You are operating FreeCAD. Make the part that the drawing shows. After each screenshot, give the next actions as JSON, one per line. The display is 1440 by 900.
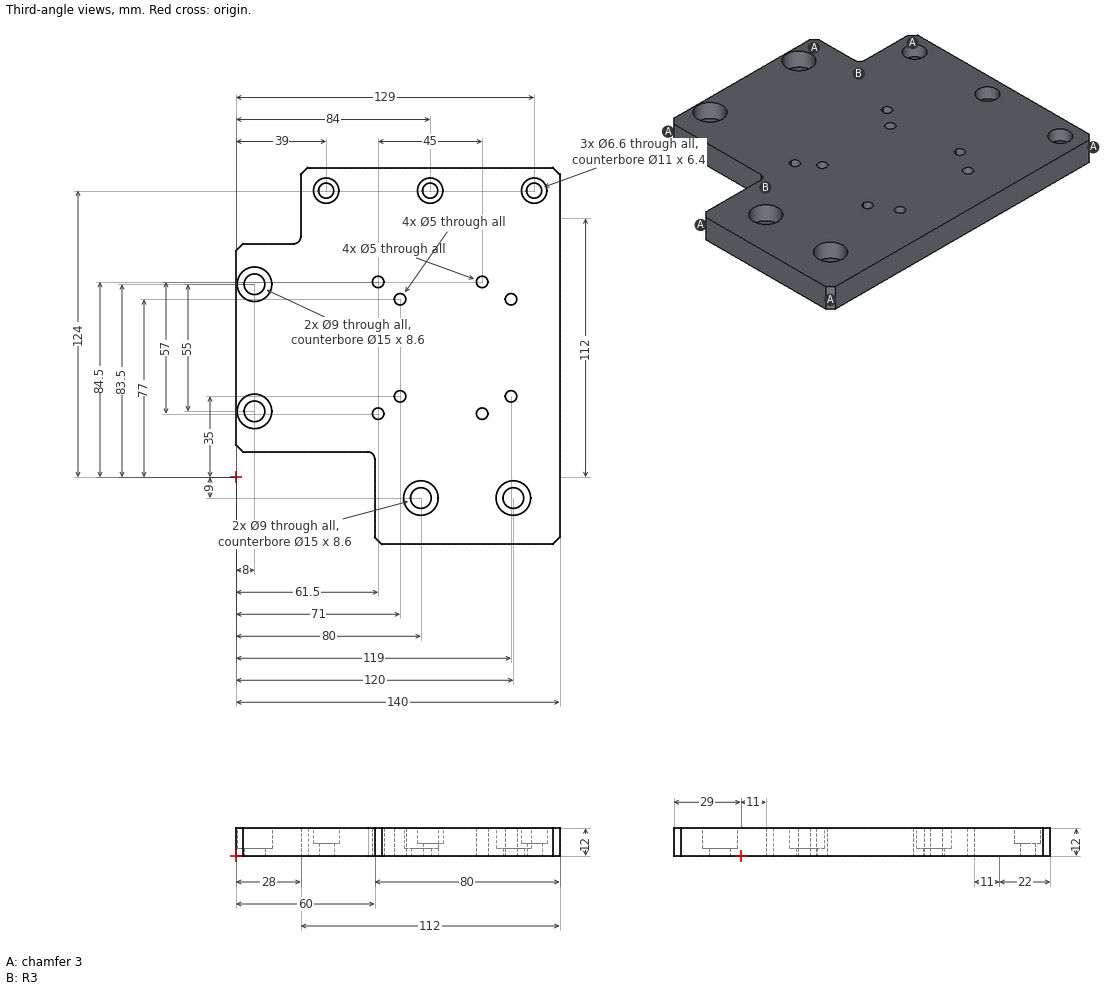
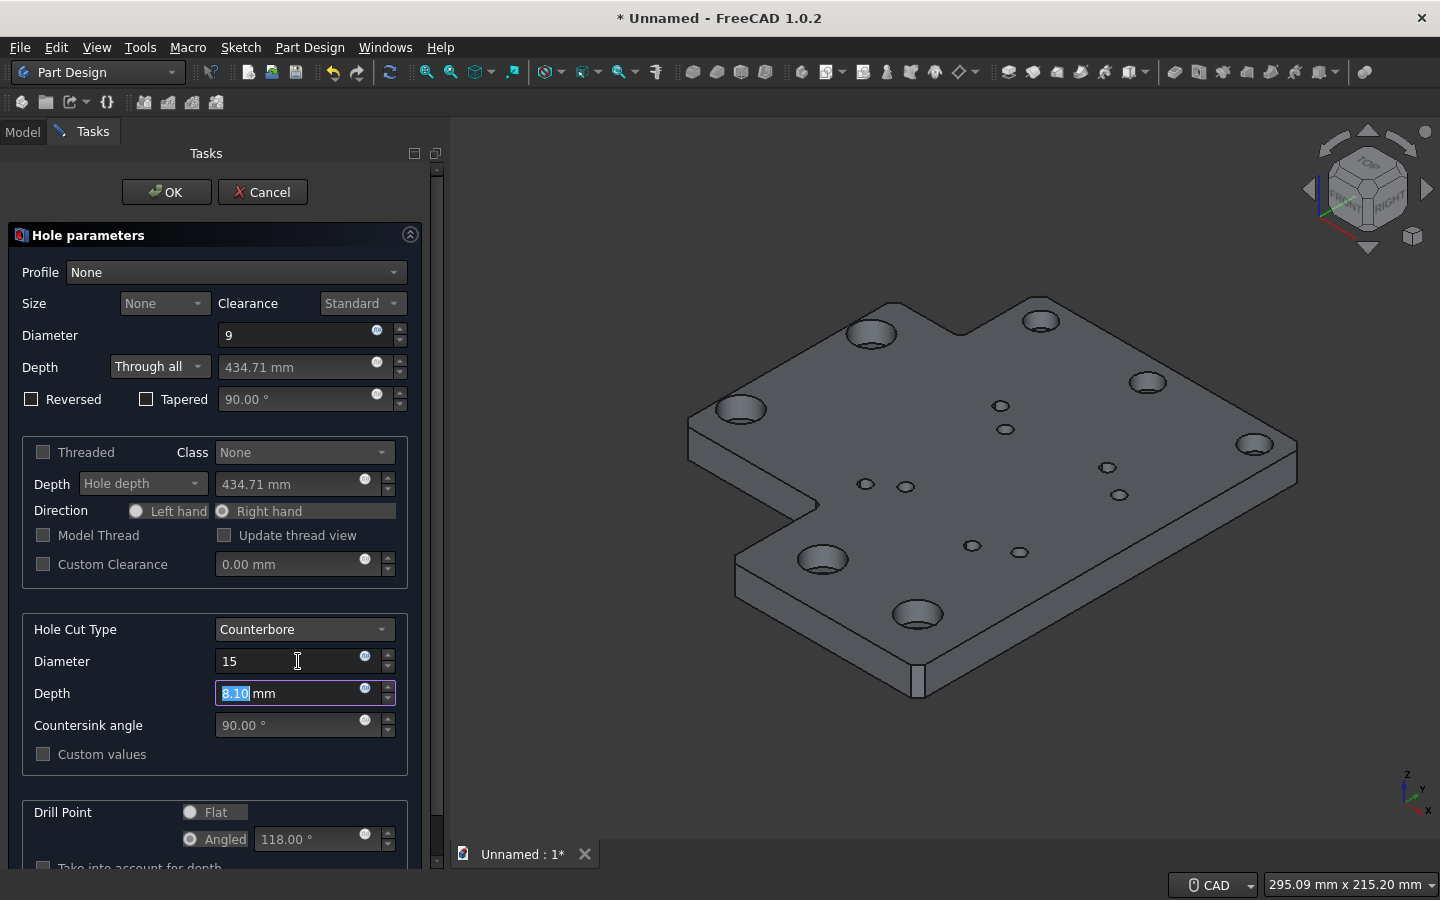
{"action": "type", "text": "8.6"}
{"action": "key", "text": "Tab"}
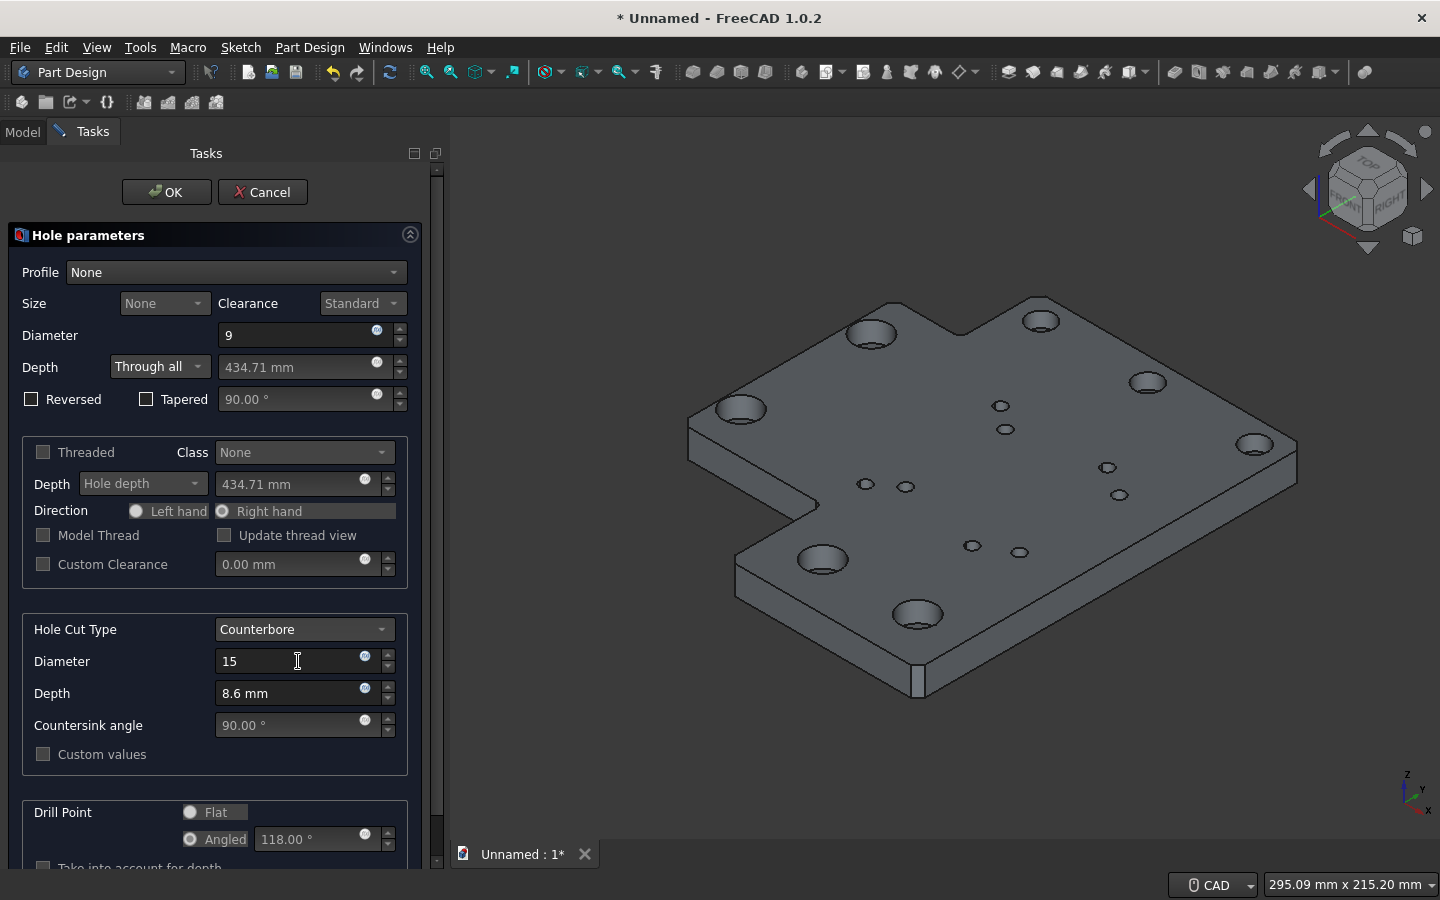
{"action": "left_click", "coordinate": [167, 192]}